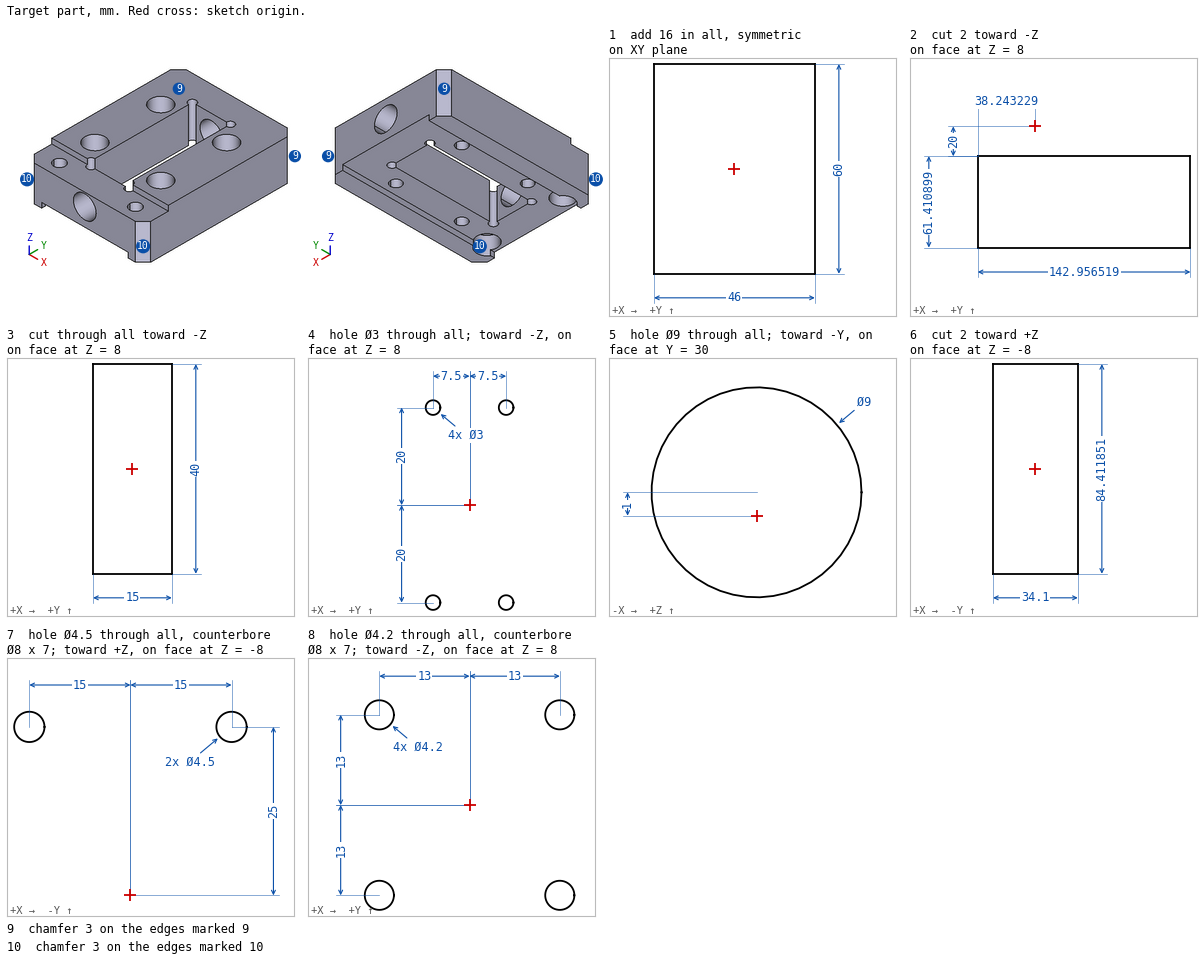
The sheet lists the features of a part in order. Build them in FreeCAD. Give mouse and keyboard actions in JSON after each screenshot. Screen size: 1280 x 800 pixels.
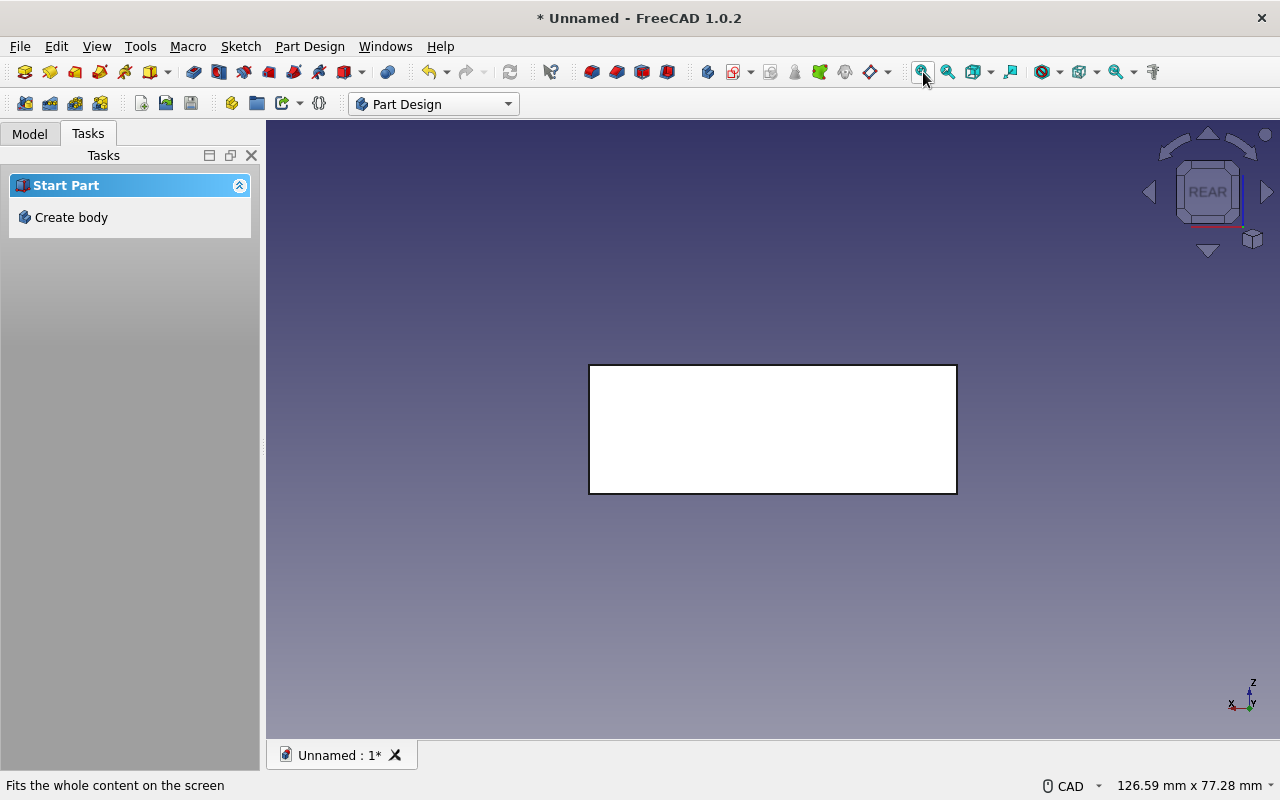
{"action": "left_click", "coordinate": [668, 429]}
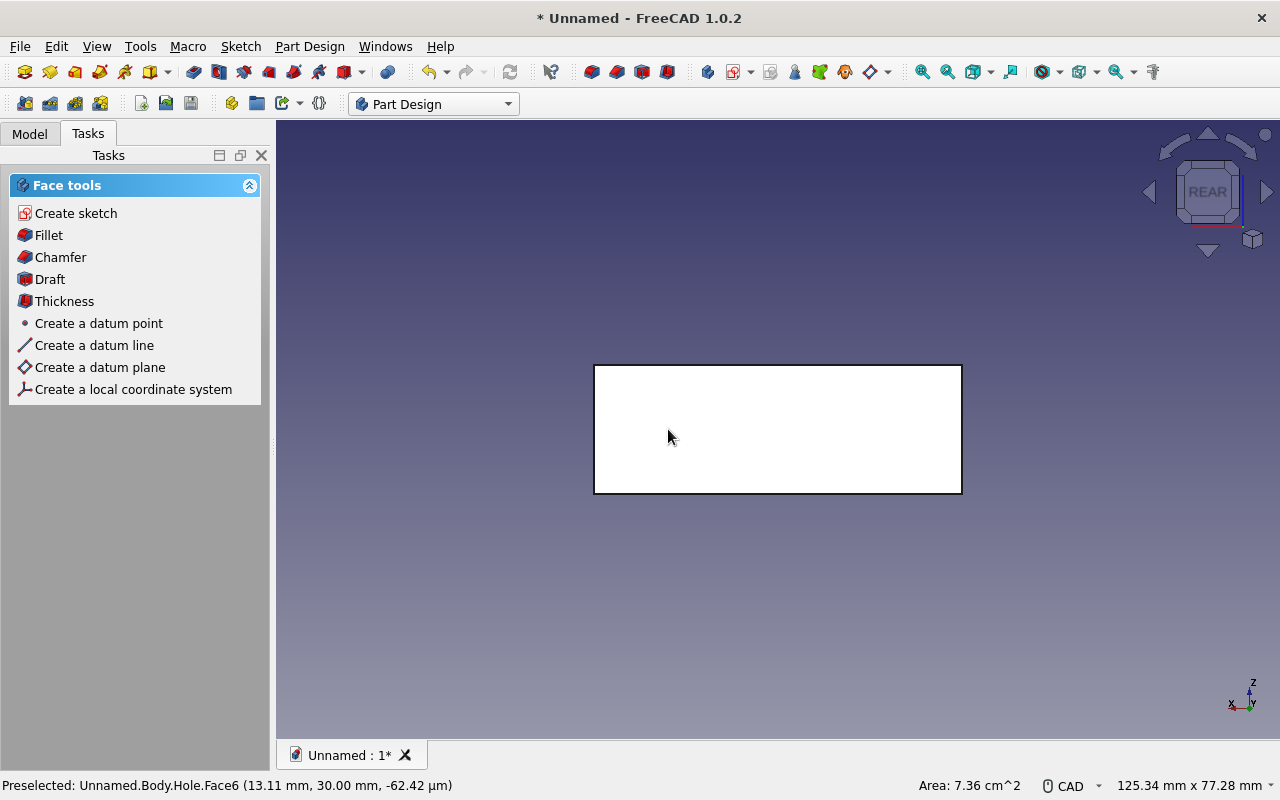
{"action": "left_click", "coordinate": [732, 72]}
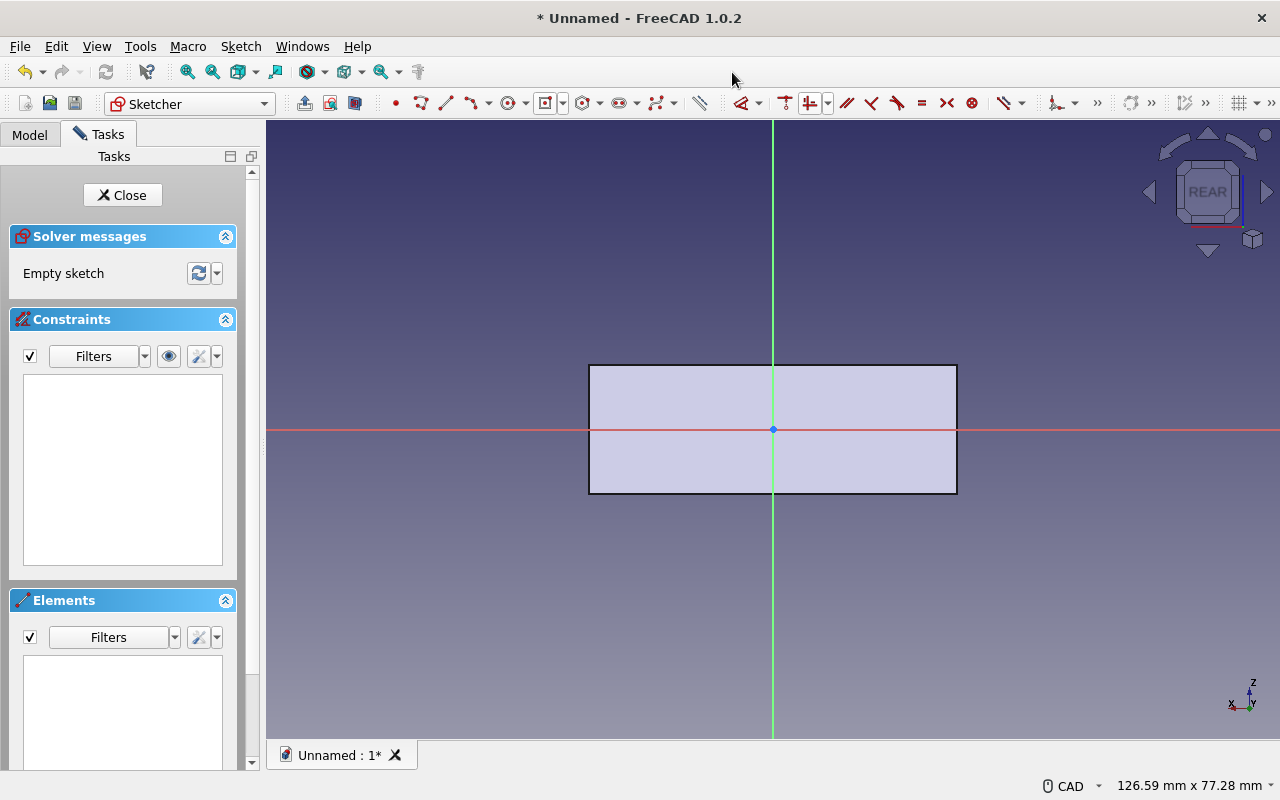
{"action": "scroll", "coordinate": [787, 420], "scroll_direction": "up", "scroll_amount": 9}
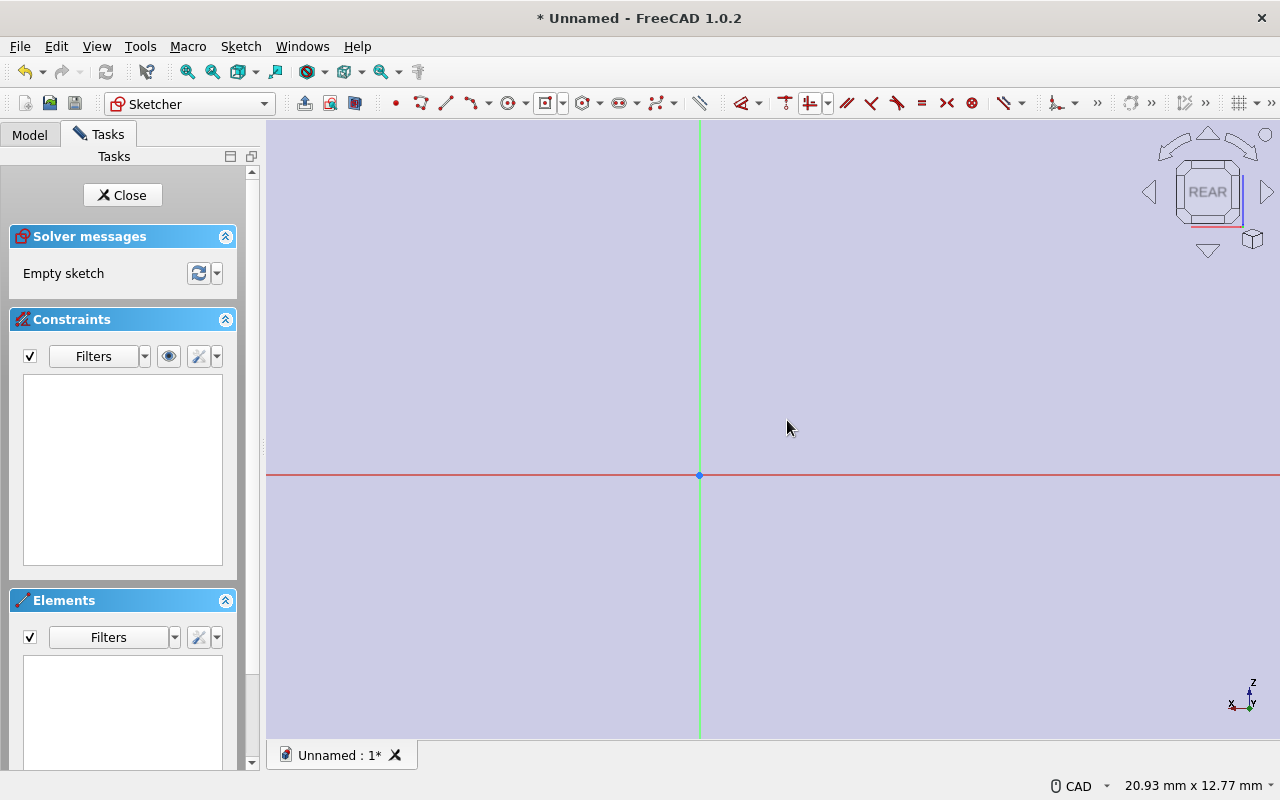
{"action": "left_click", "coordinate": [508, 104]}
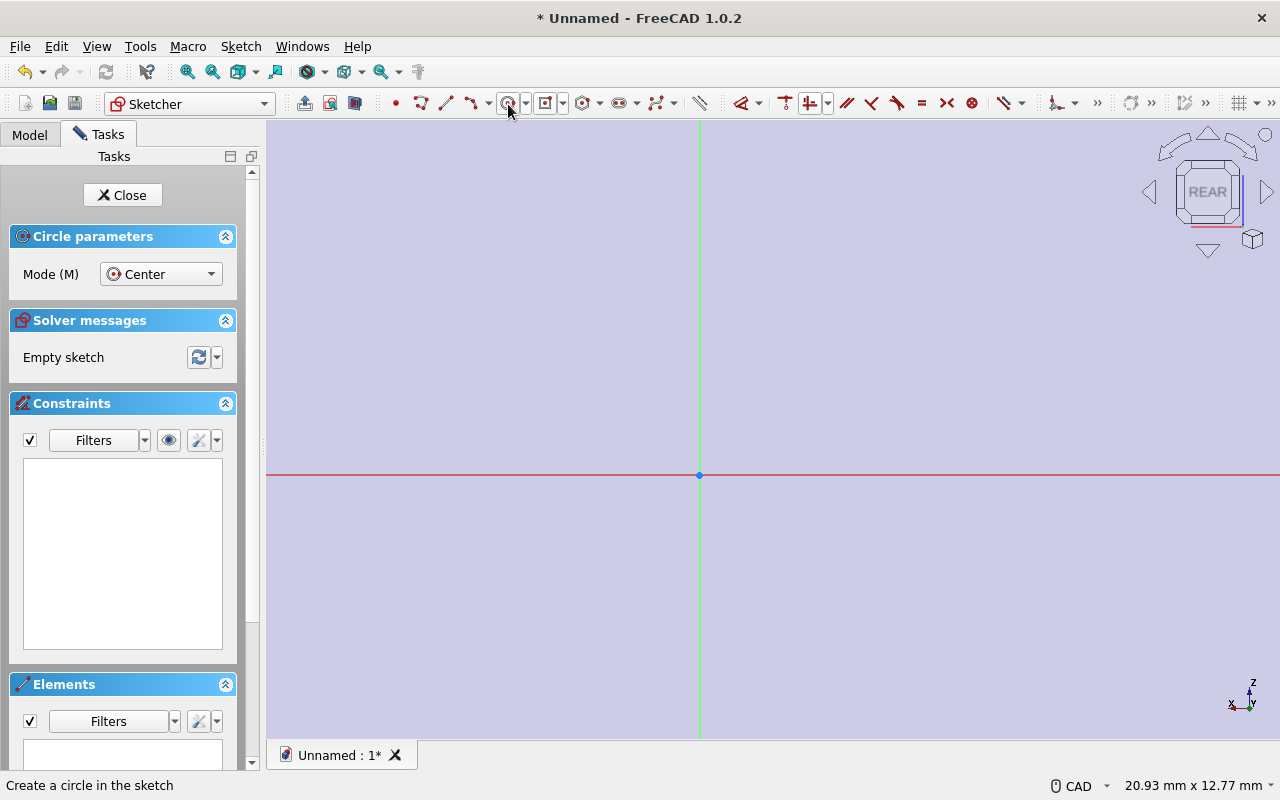
{"action": "left_click", "coordinate": [700, 427]}
{"action": "left_click", "coordinate": [854, 272]}
{"action": "key", "text": "Escape"}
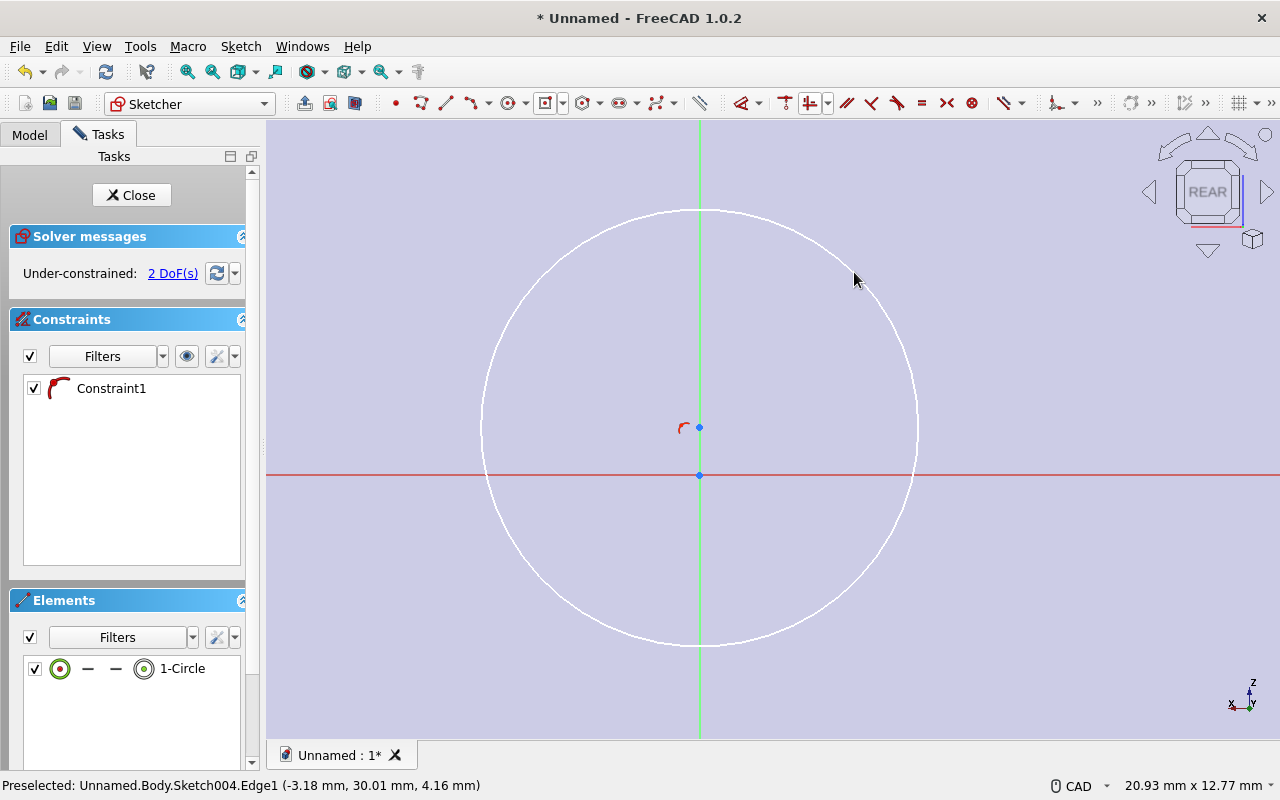
{"action": "left_click", "coordinate": [740, 104]}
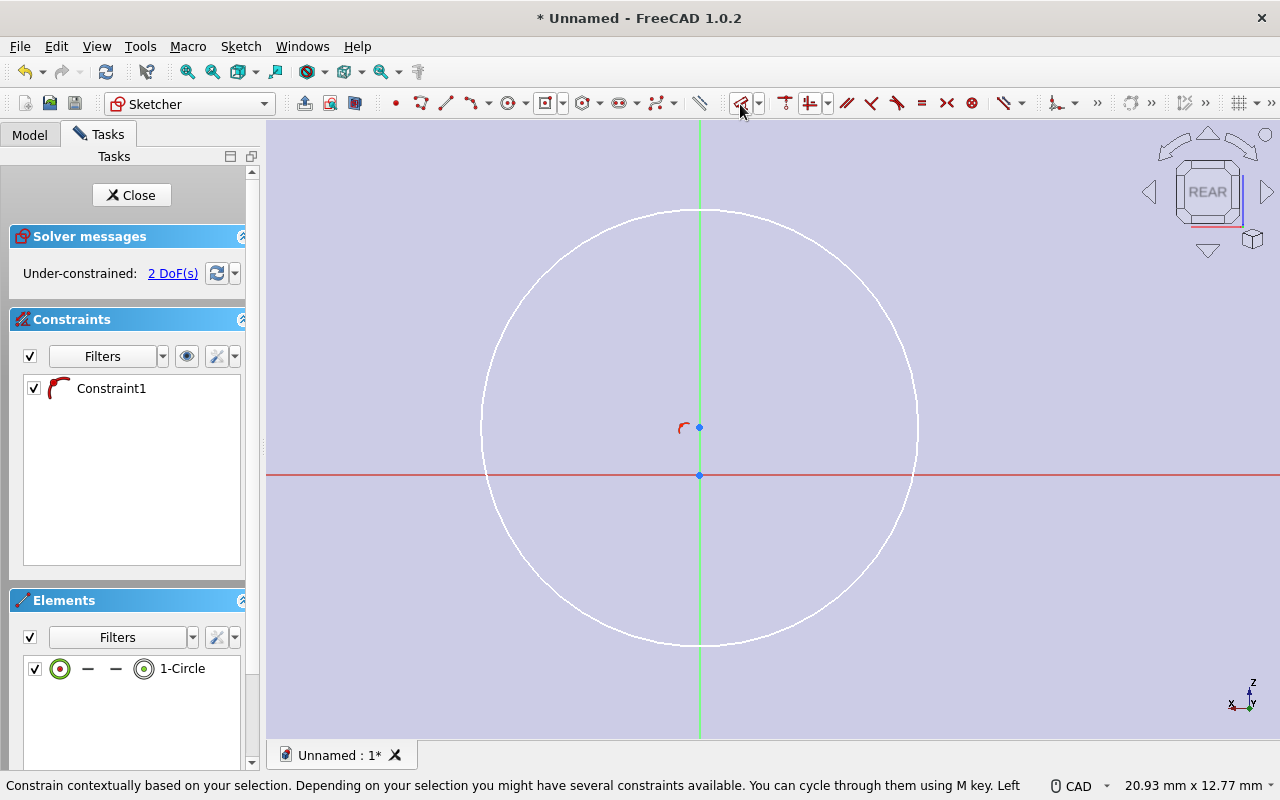
{"action": "left_click", "coordinate": [854, 273]}
{"action": "left_click", "coordinate": [877, 250]}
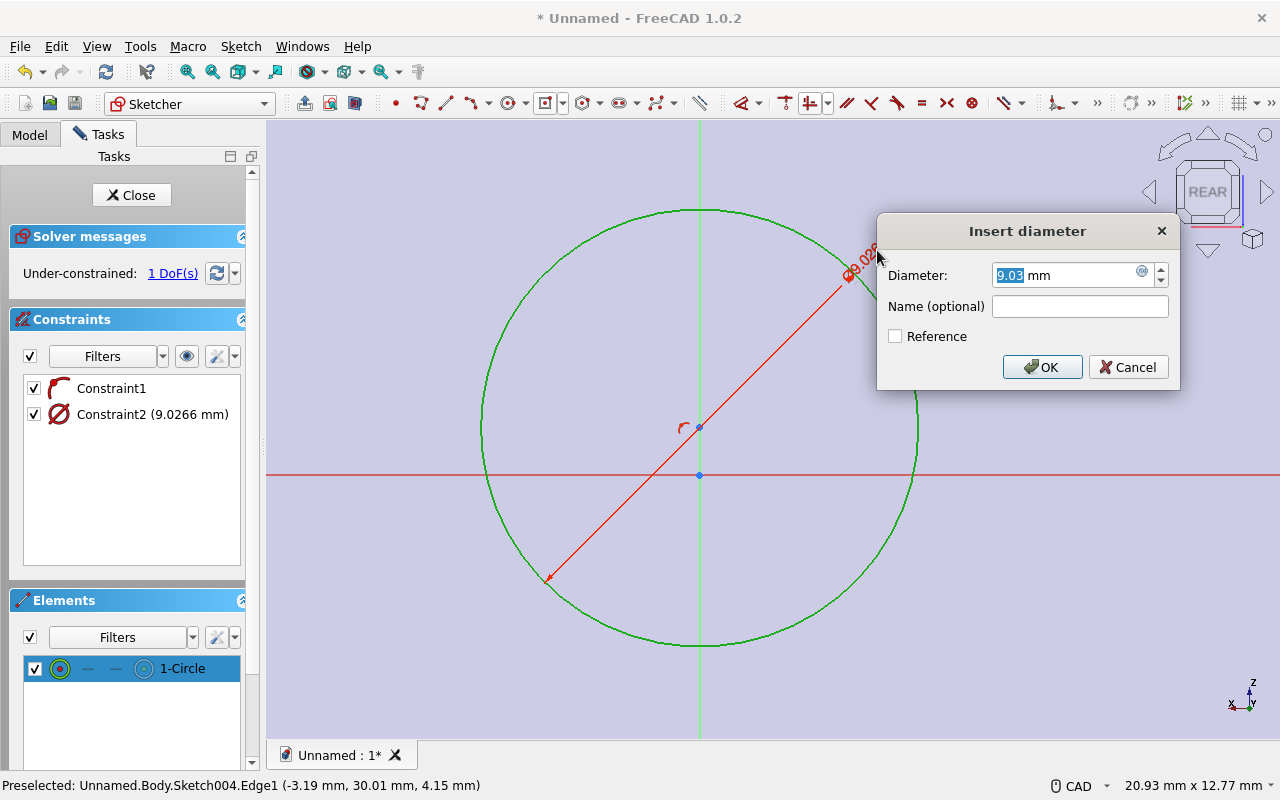
{"action": "type", "text": "9"}
{"action": "key", "text": "Return"}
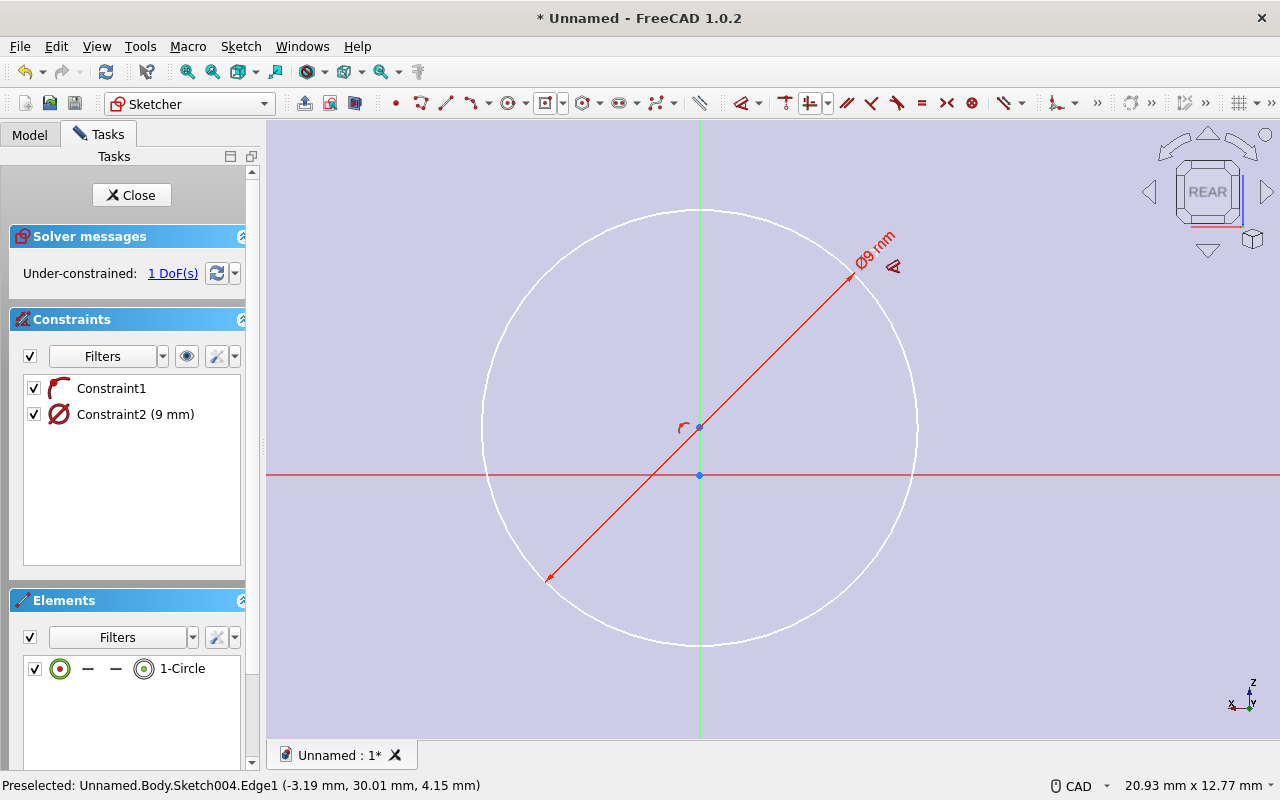
{"action": "left_click", "coordinate": [700, 428]}
{"action": "left_click", "coordinate": [734, 452]}